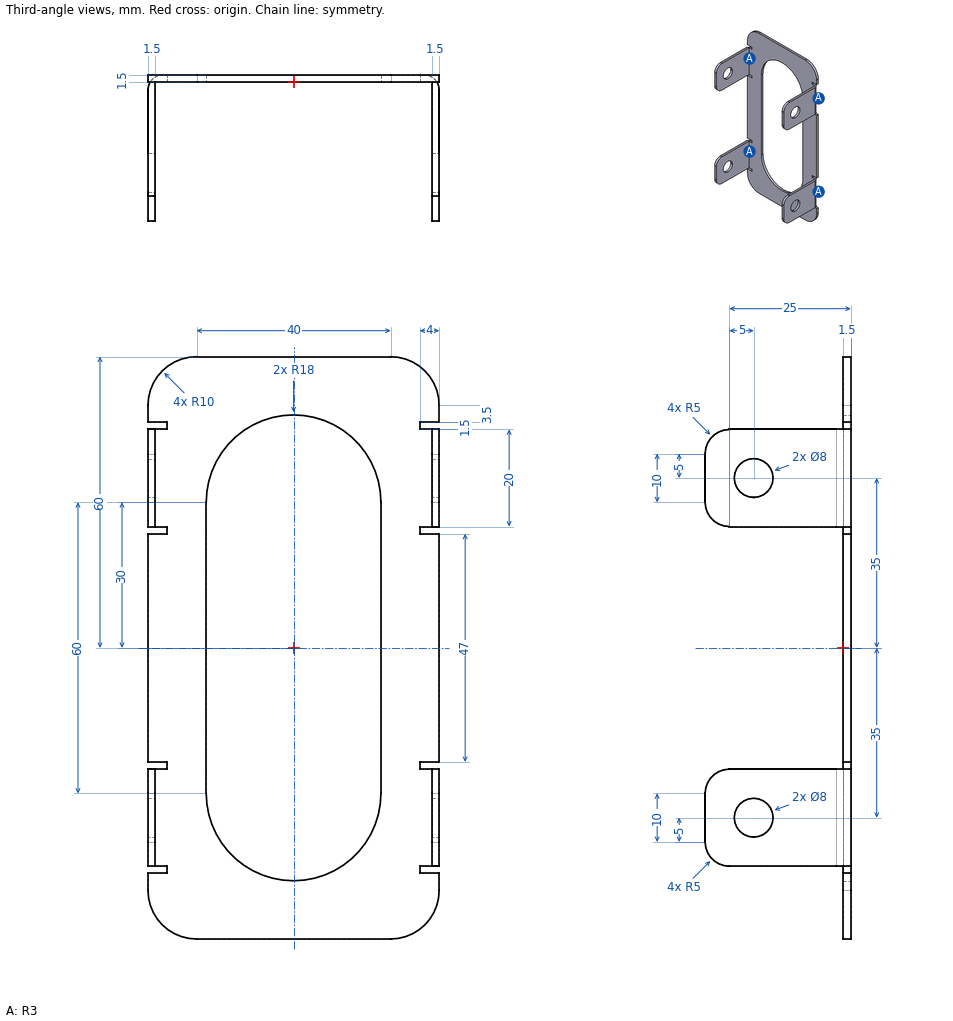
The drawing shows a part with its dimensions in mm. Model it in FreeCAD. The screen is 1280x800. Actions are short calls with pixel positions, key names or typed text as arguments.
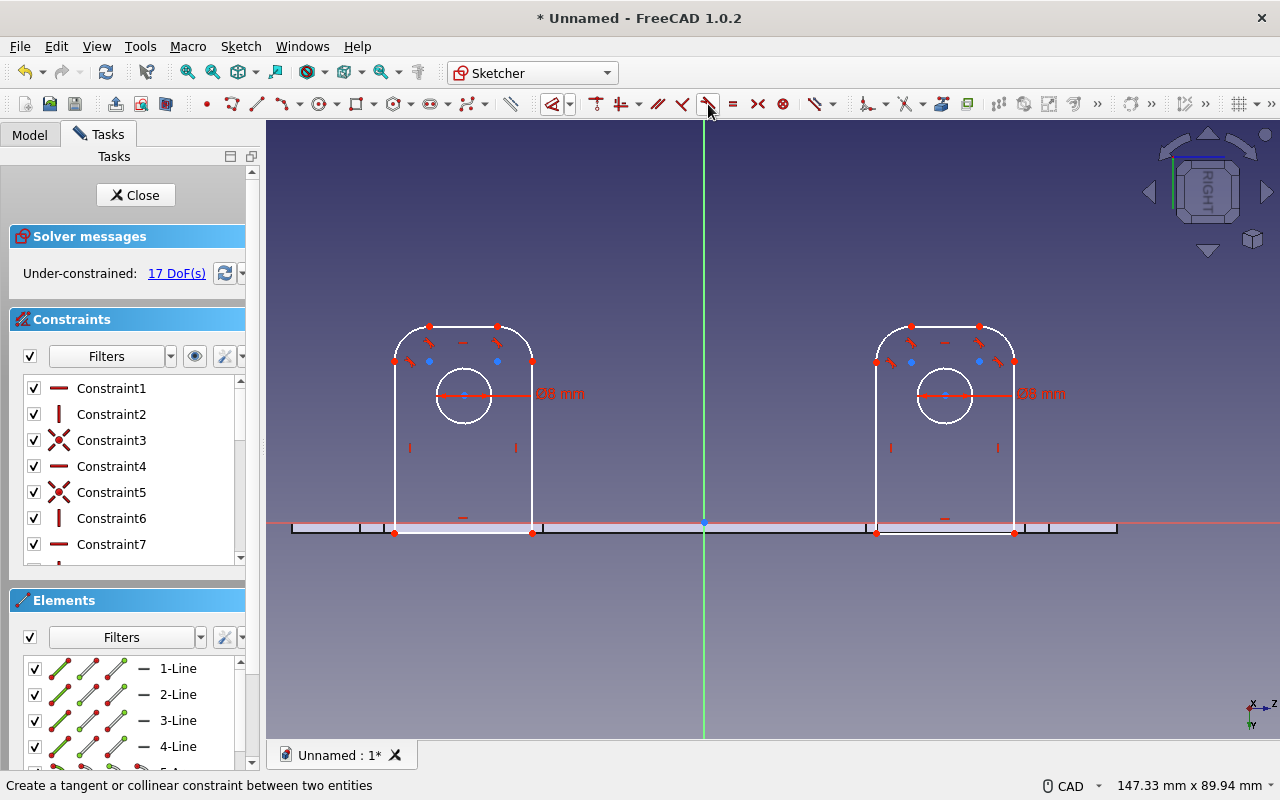
click(532, 482)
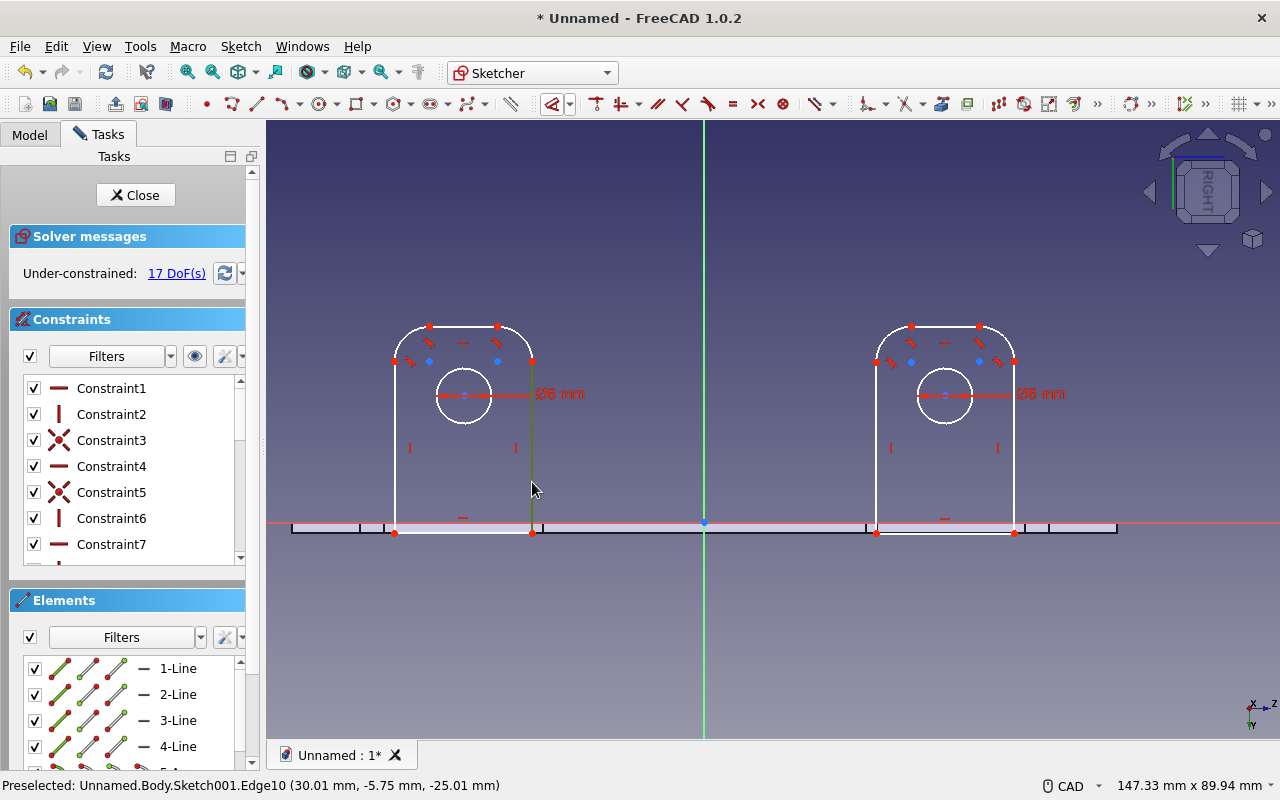
click(528, 346)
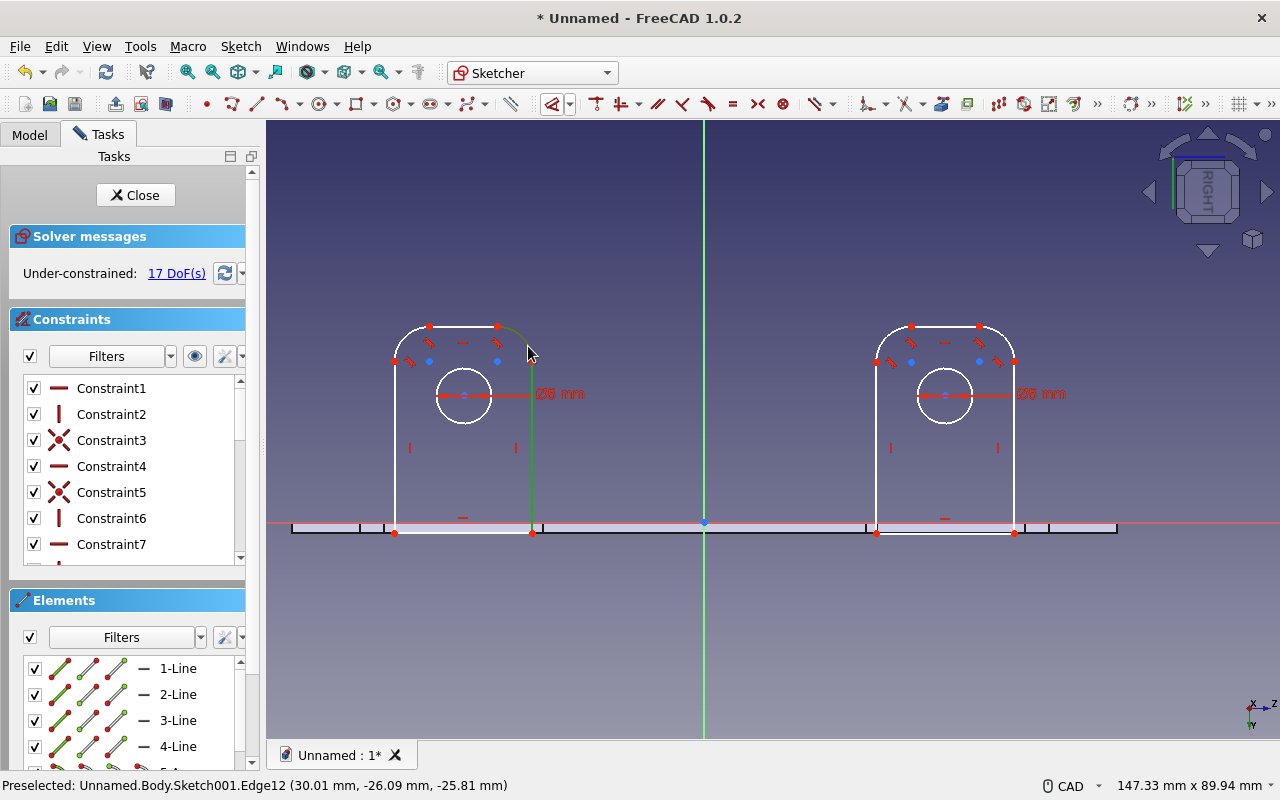
click(708, 104)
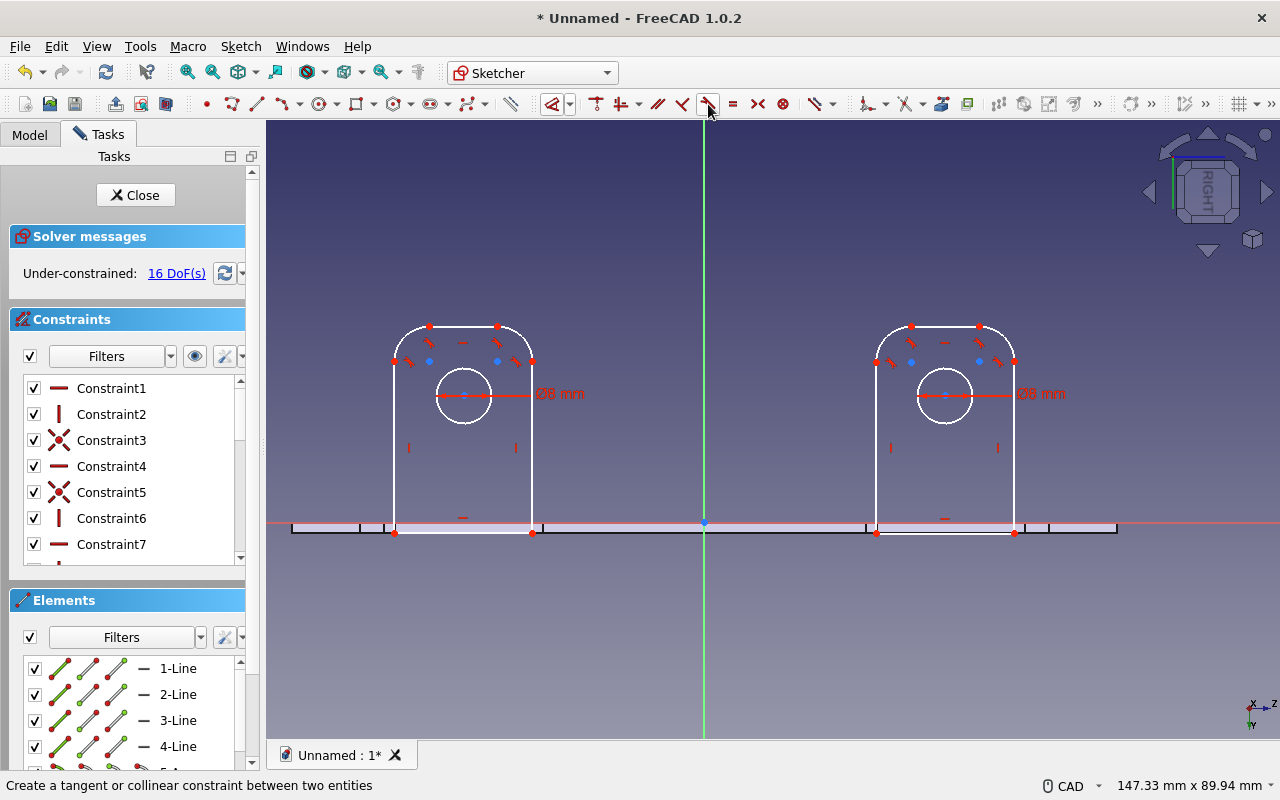
click(896, 331)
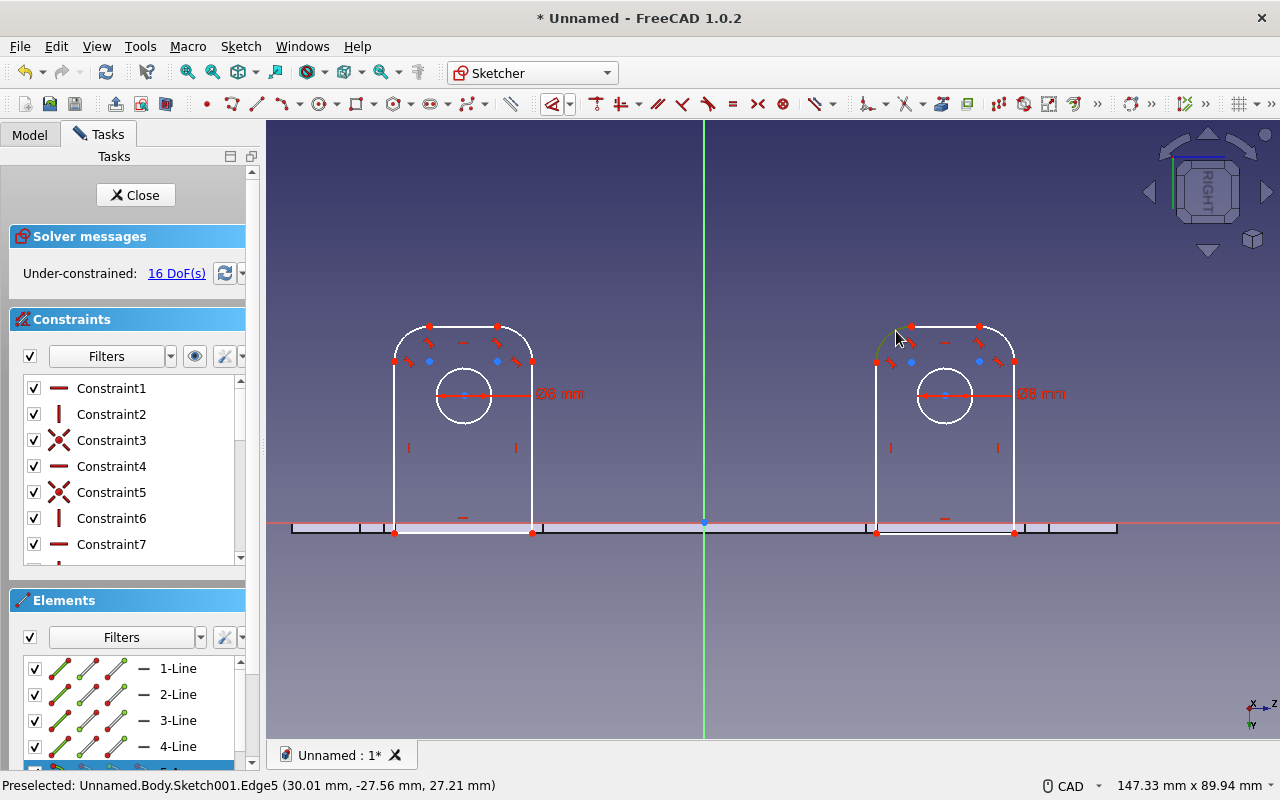
click(1011, 346)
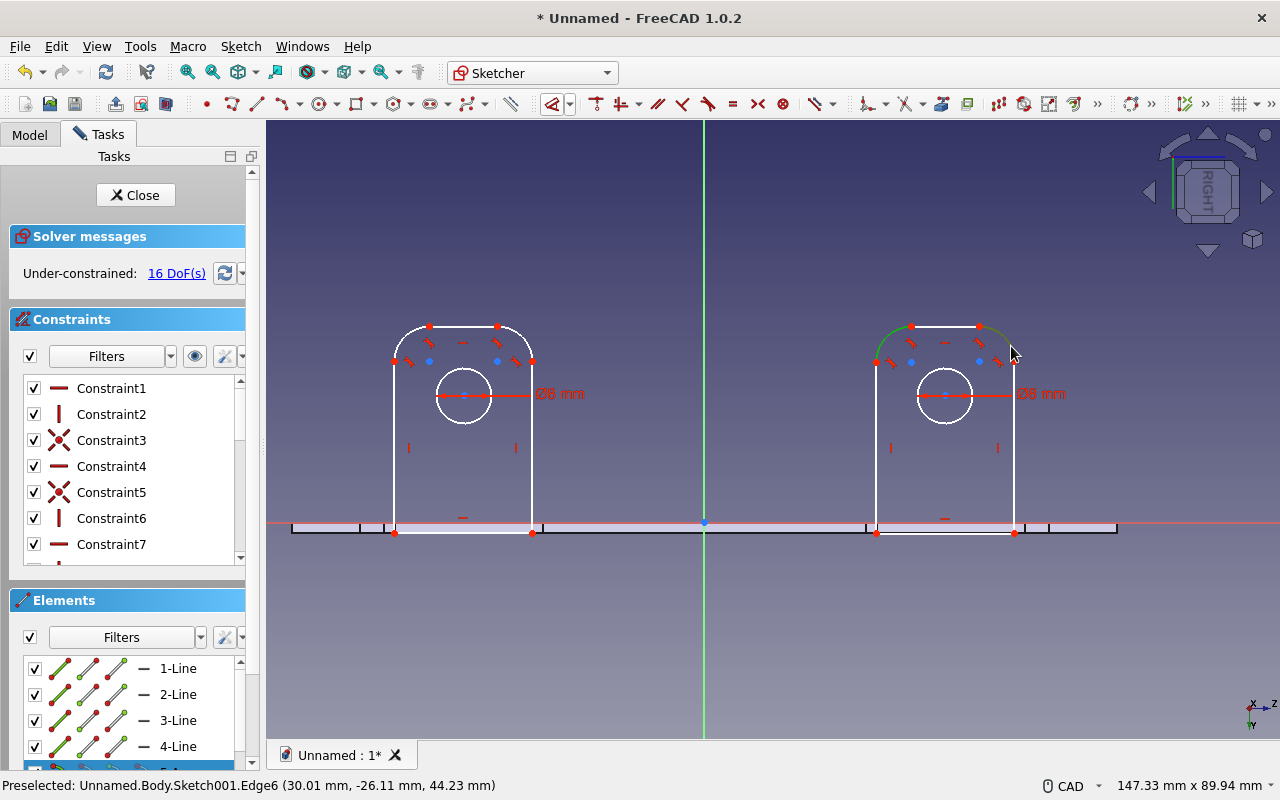
click(414, 331)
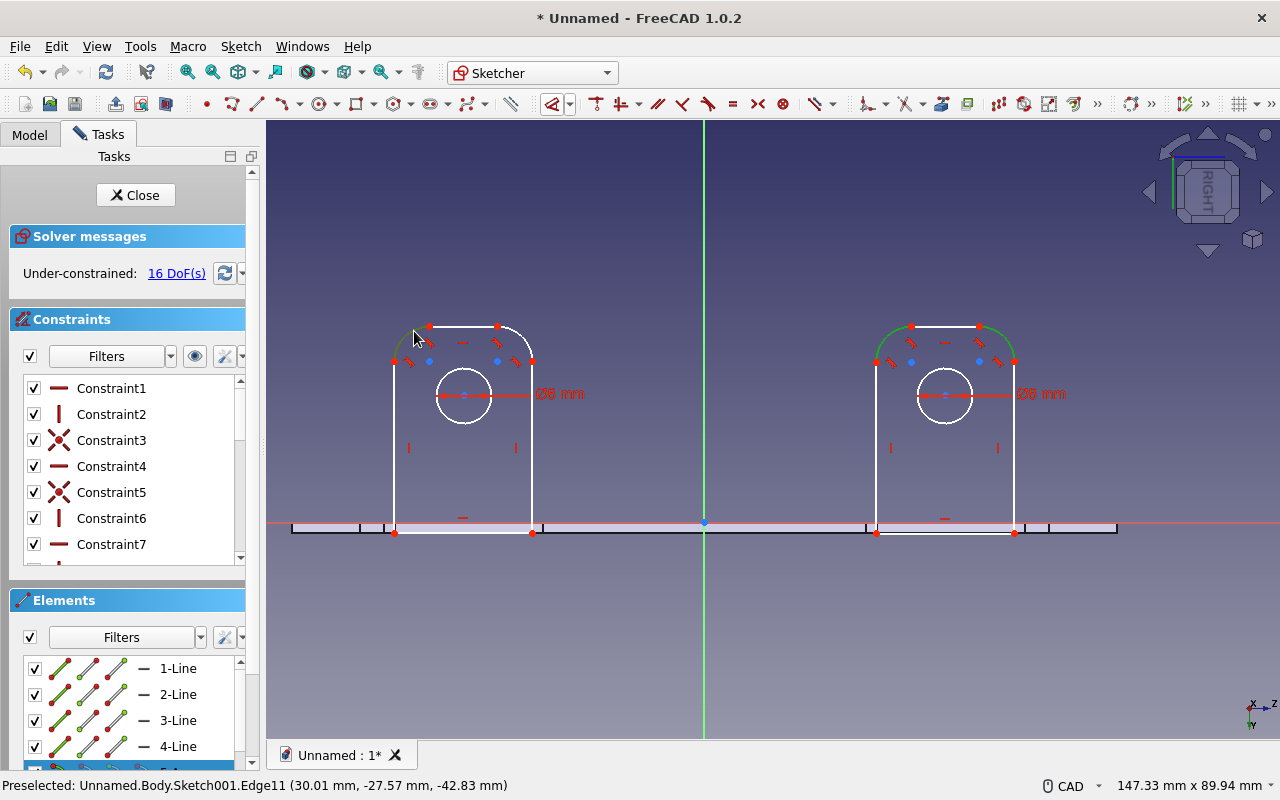
click(529, 346)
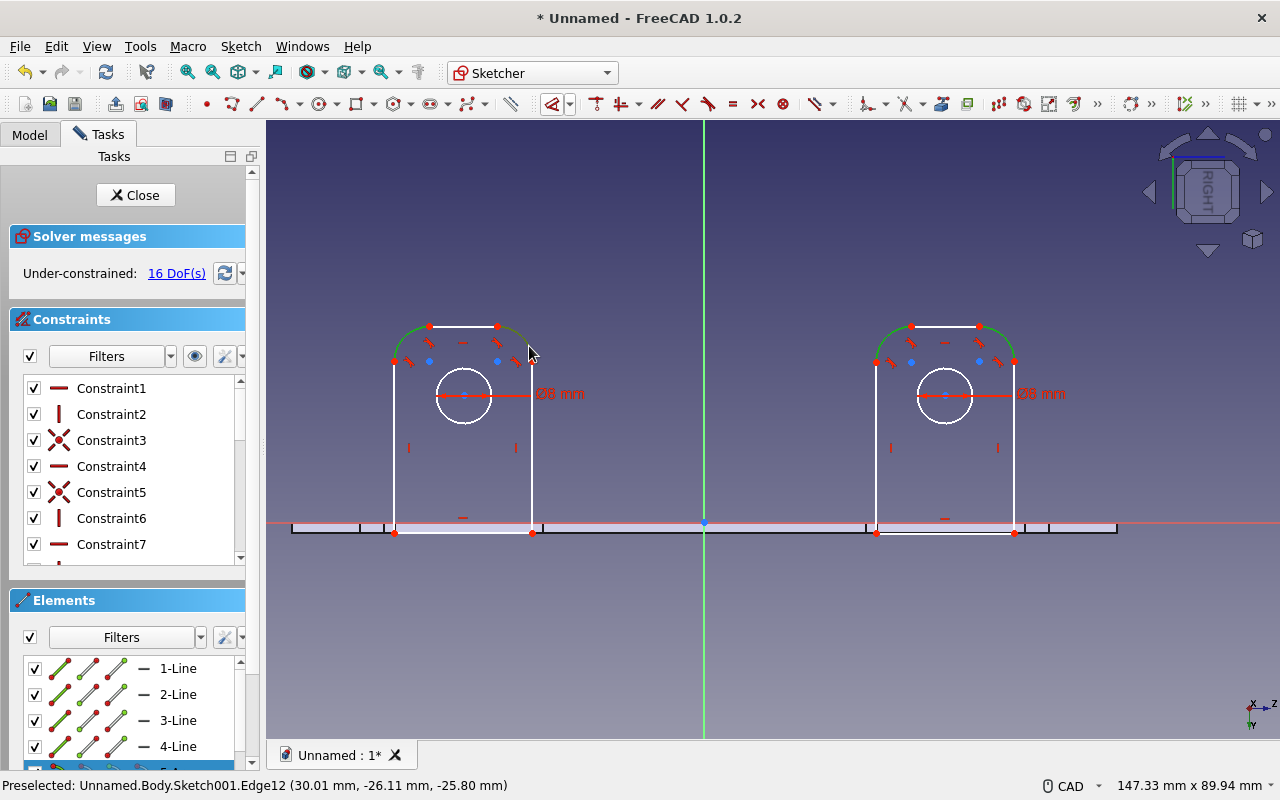
click(733, 104)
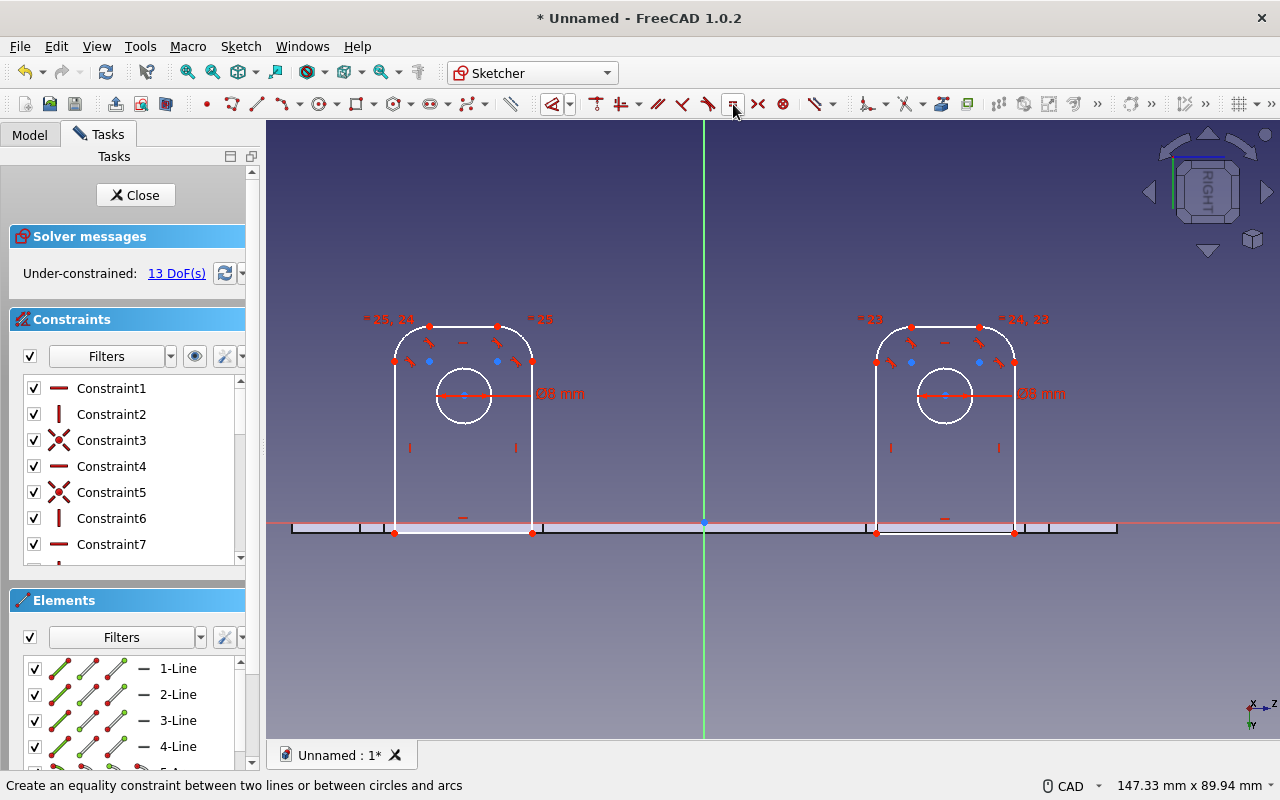
click(980, 362)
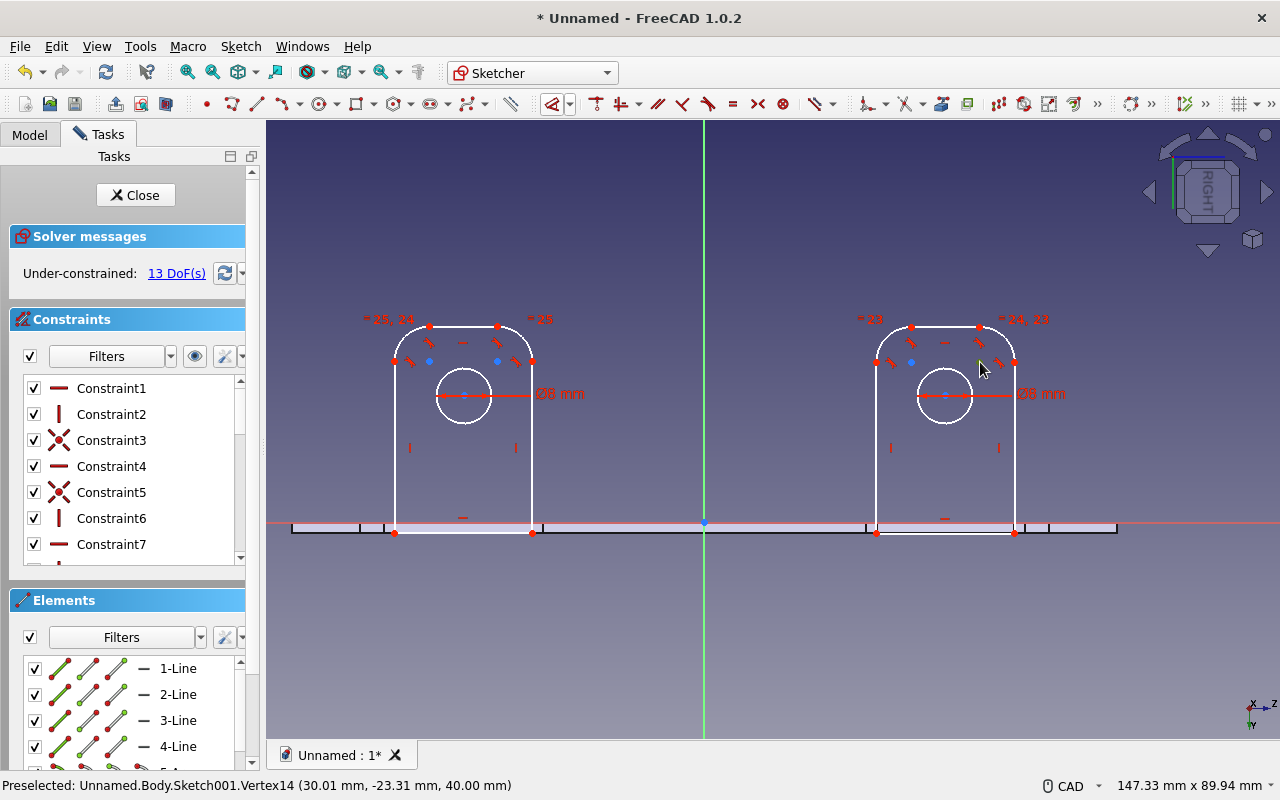
click(430, 362)